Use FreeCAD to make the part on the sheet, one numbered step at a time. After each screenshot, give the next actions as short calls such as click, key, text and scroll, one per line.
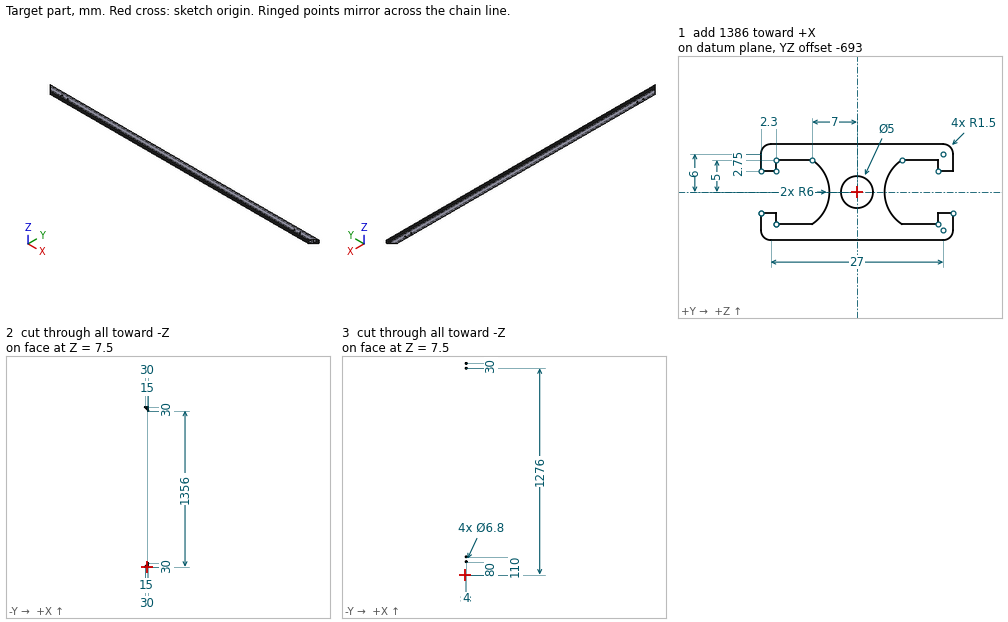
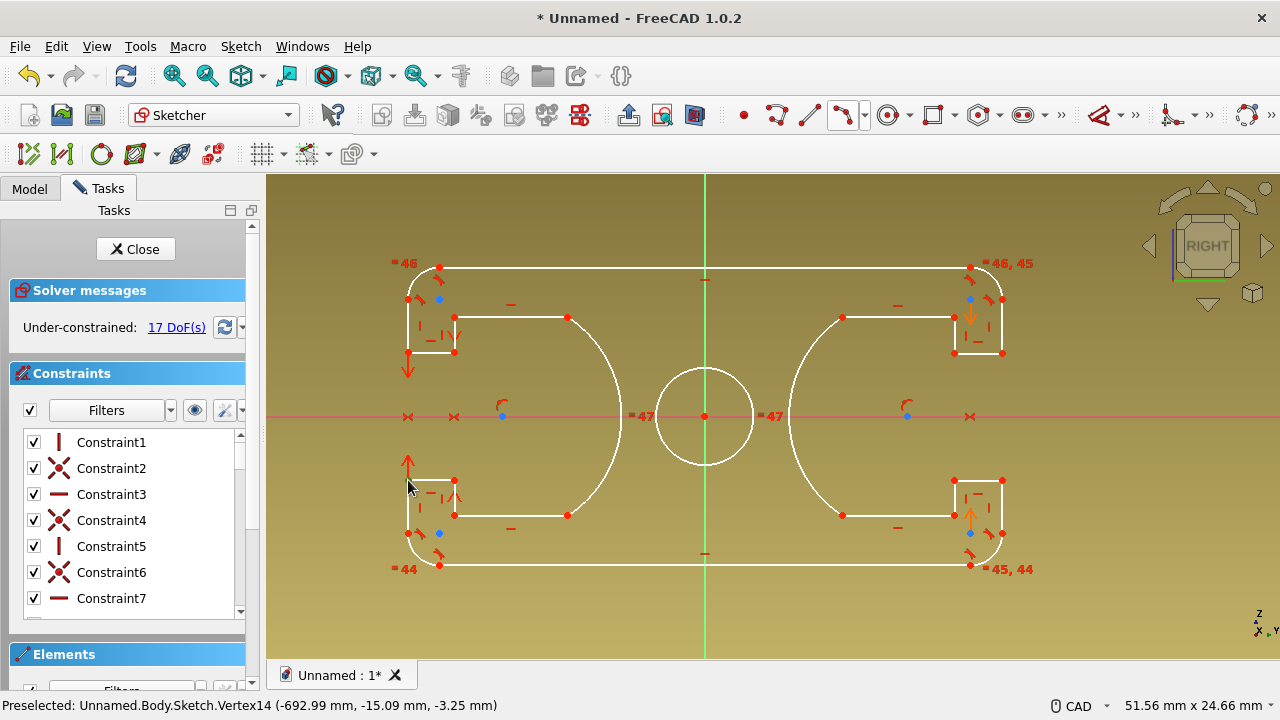
click(1002, 481)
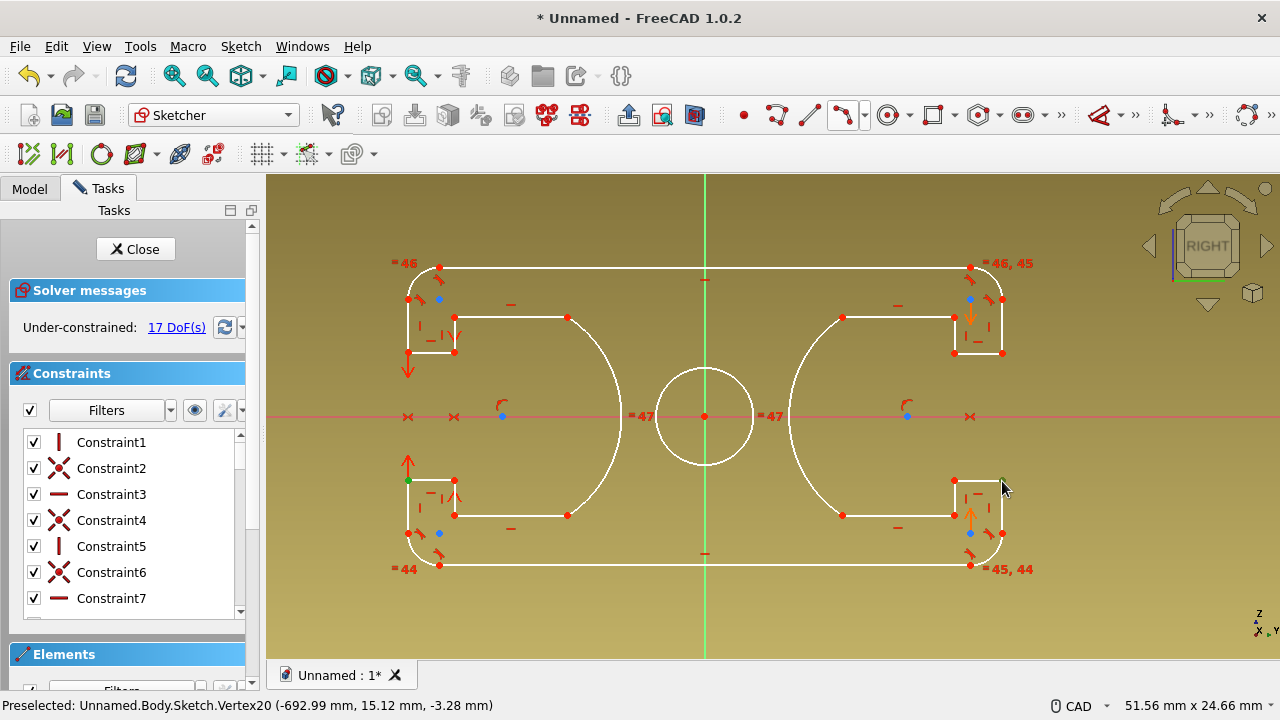
click(705, 600)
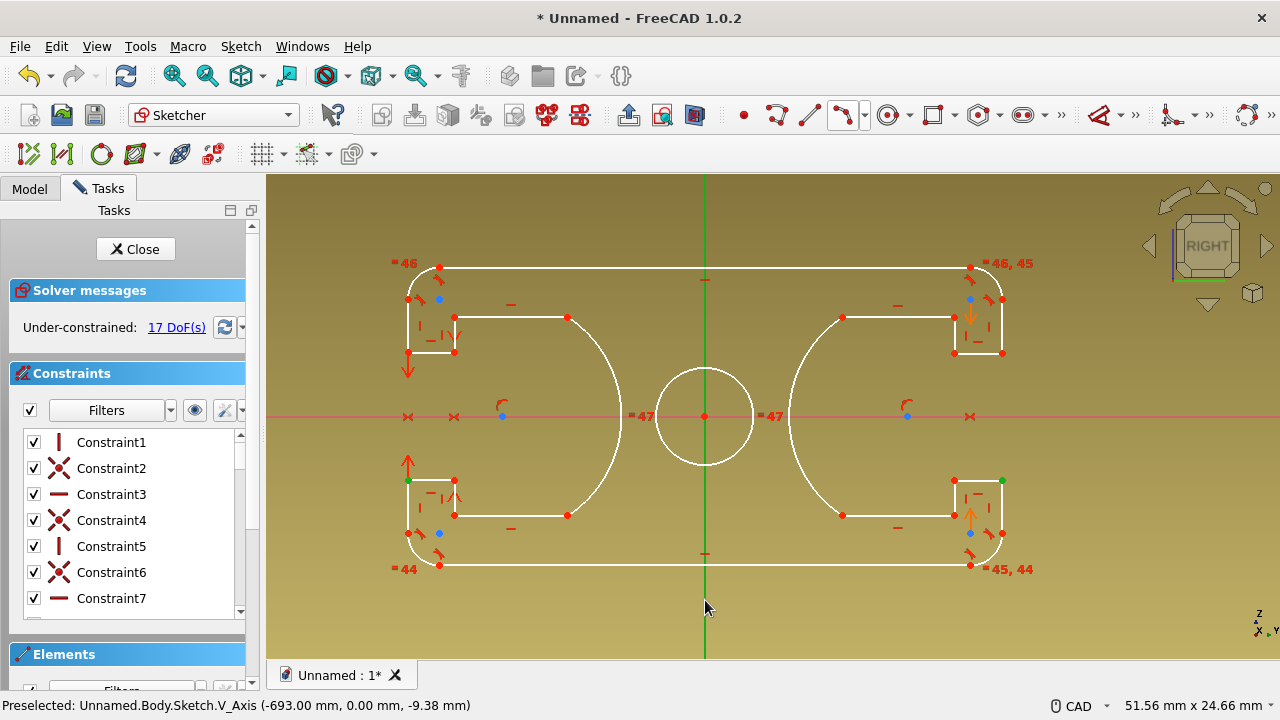
key(s)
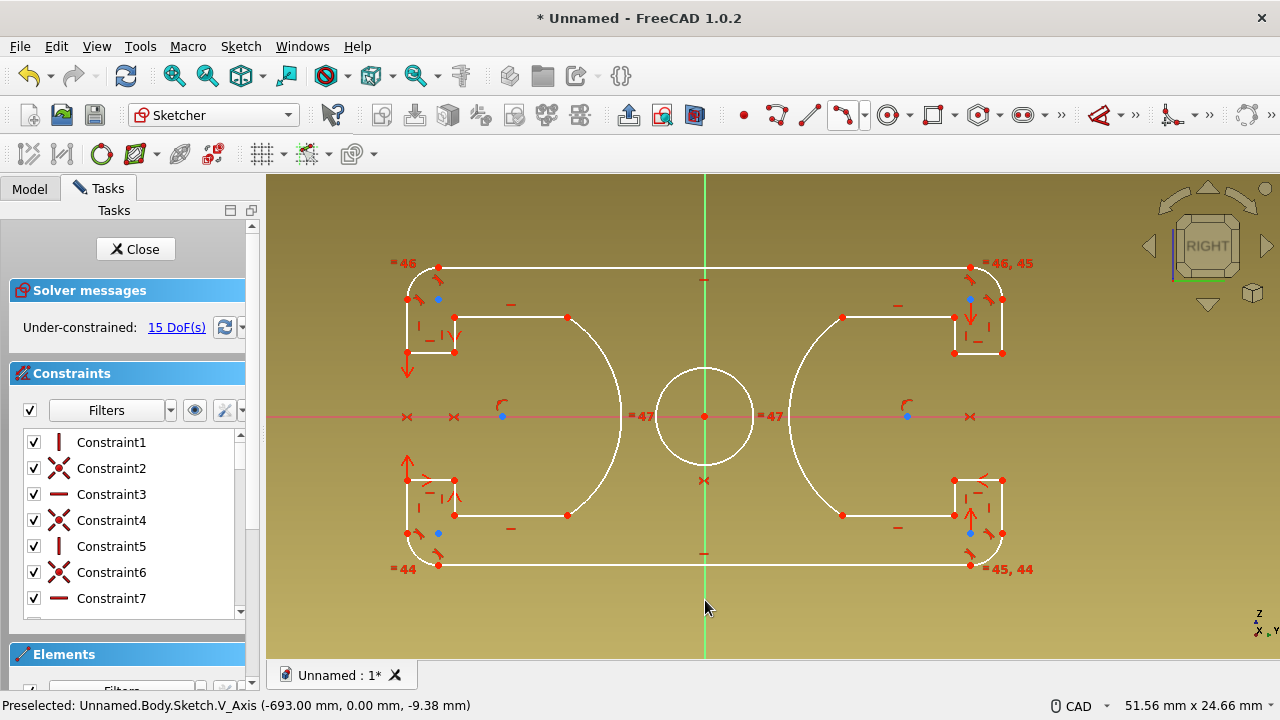
click(455, 516)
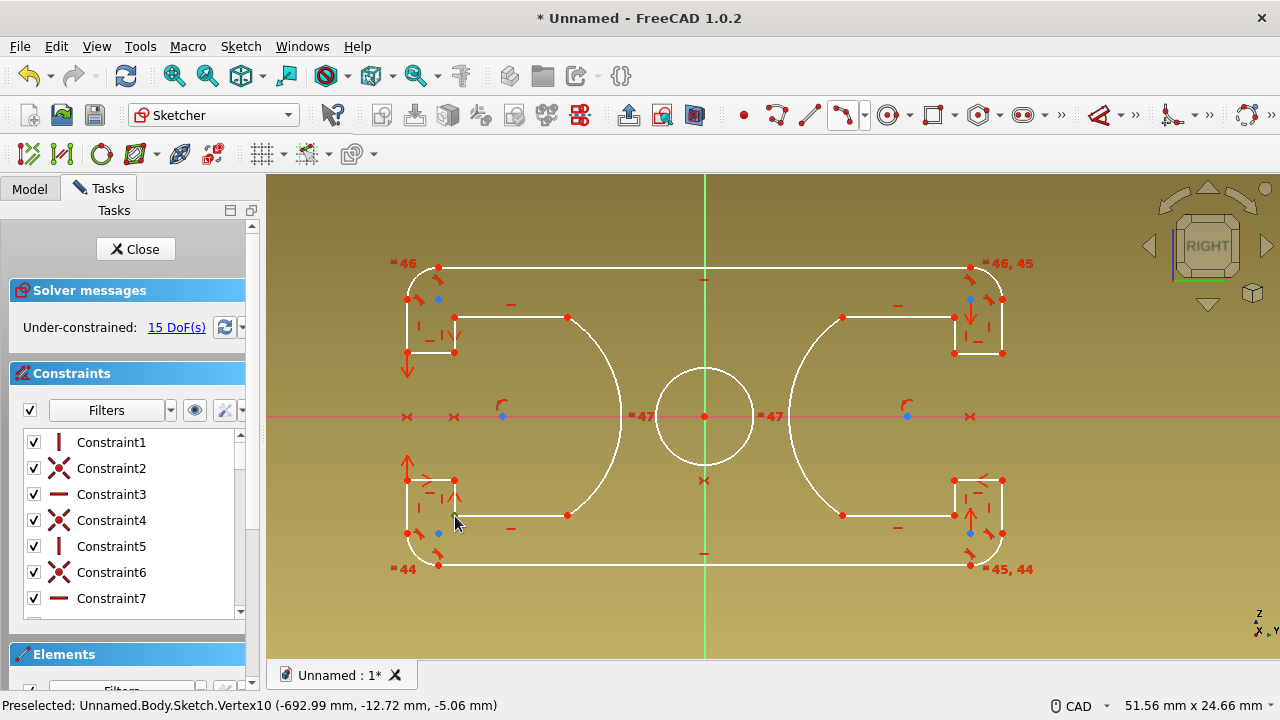
click(955, 516)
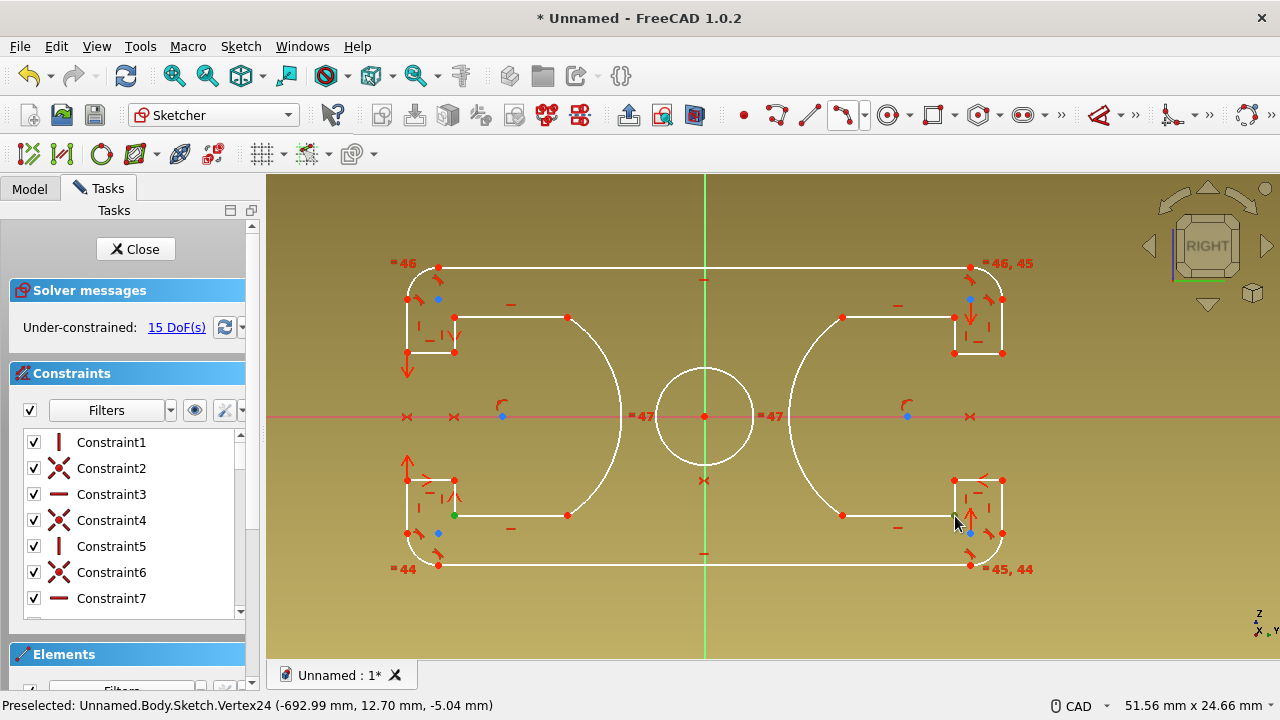
click(705, 600)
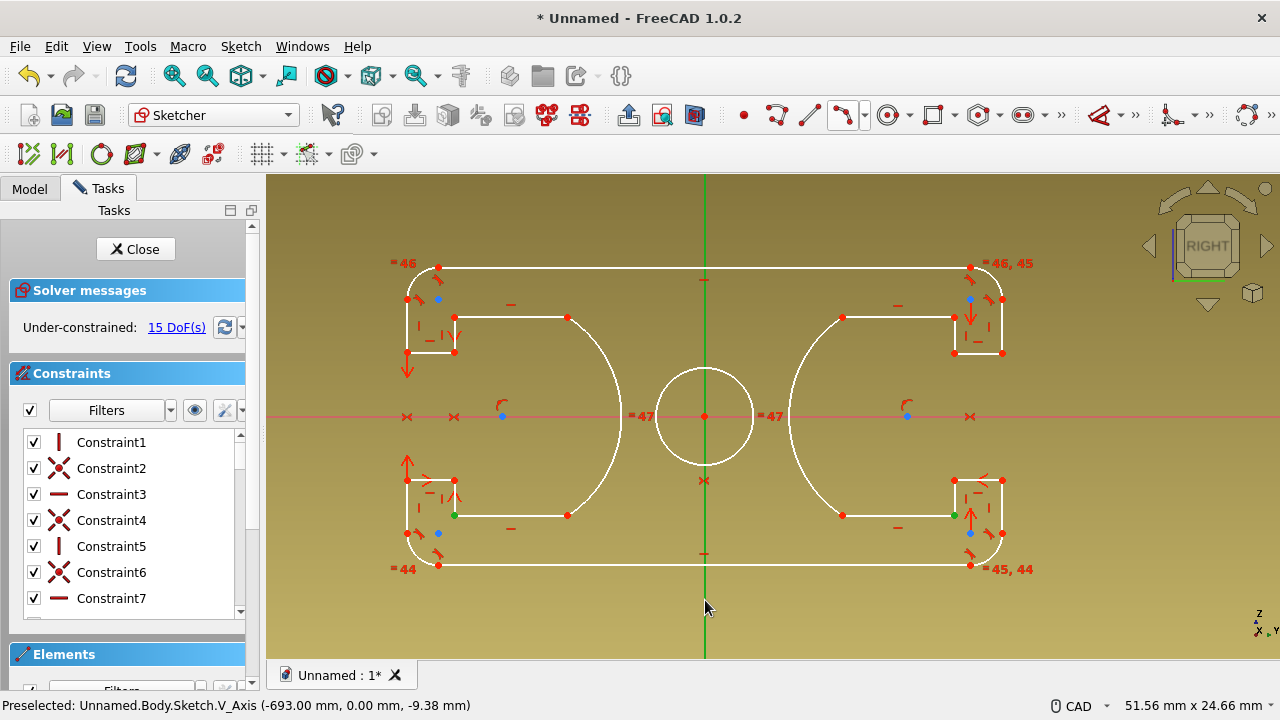
key(s)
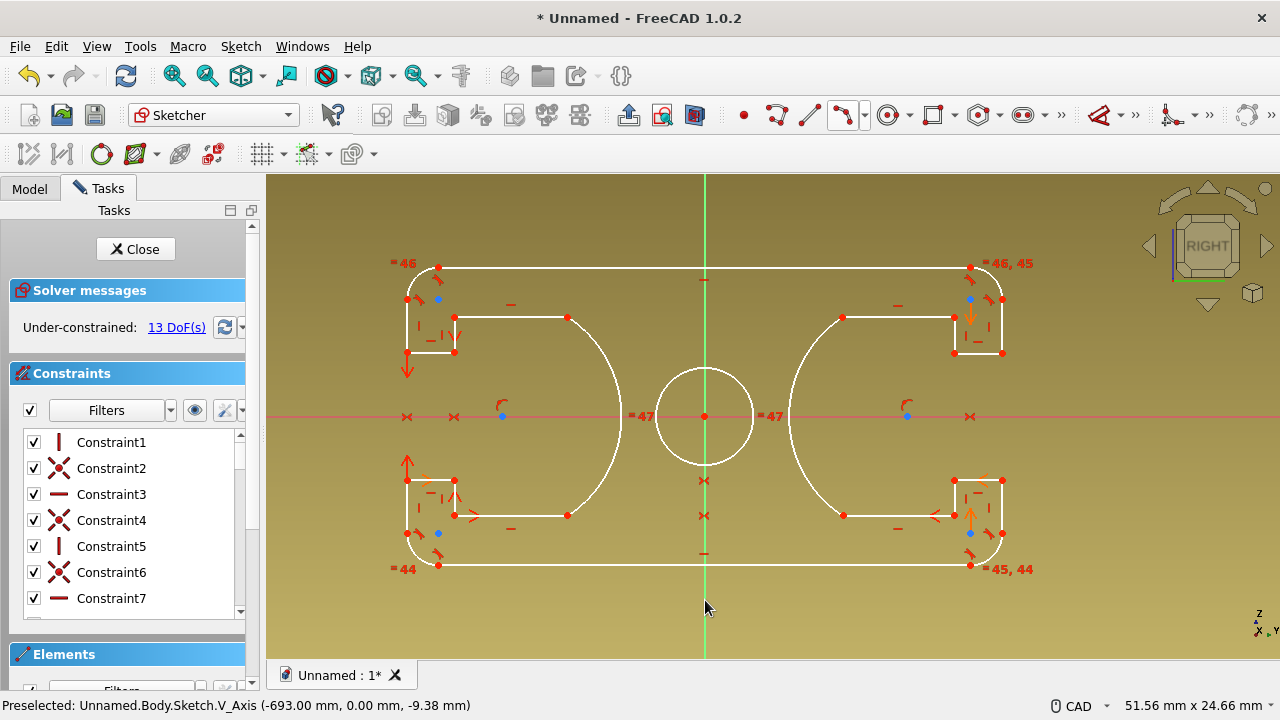
click(568, 317)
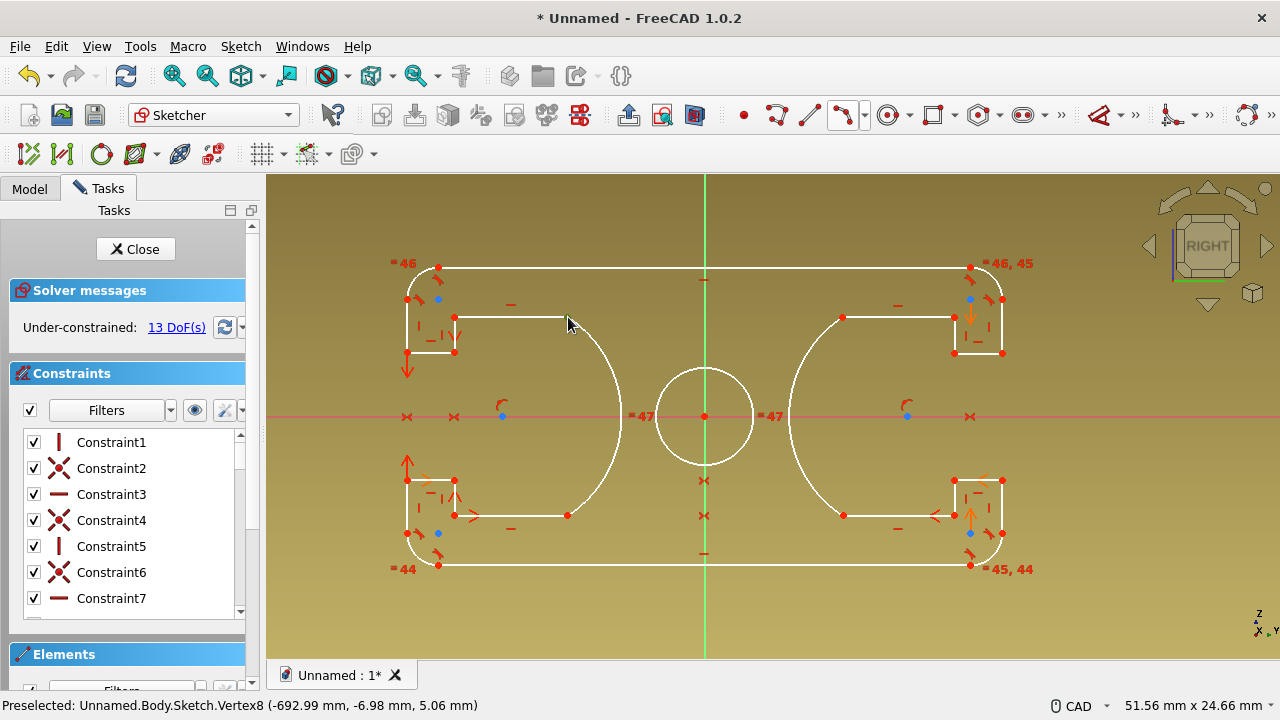
click(843, 317)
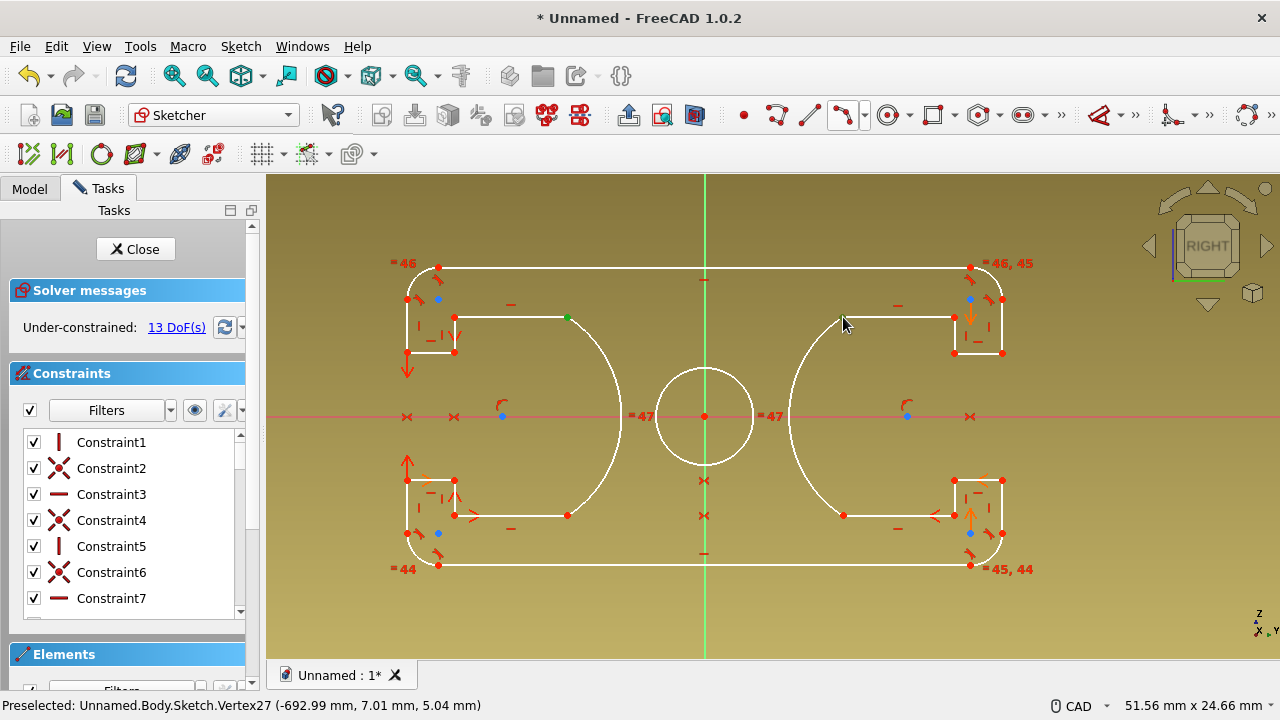
click(705, 600)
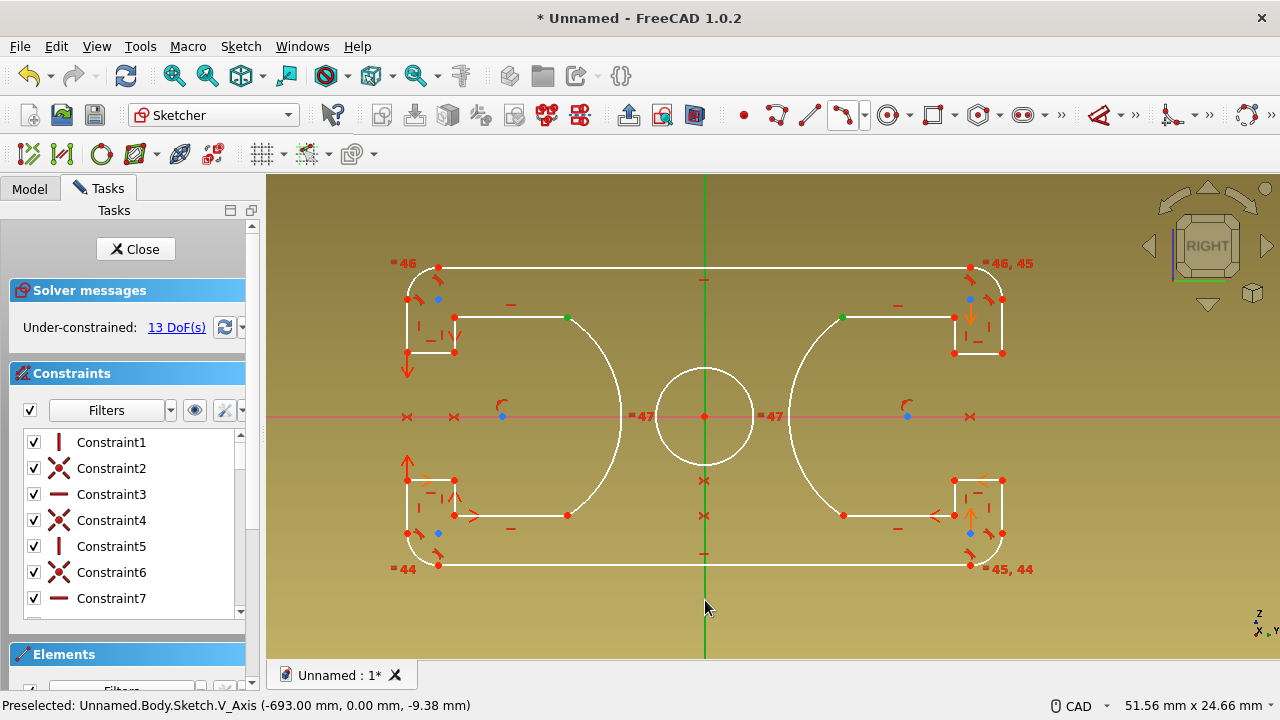
key(s)